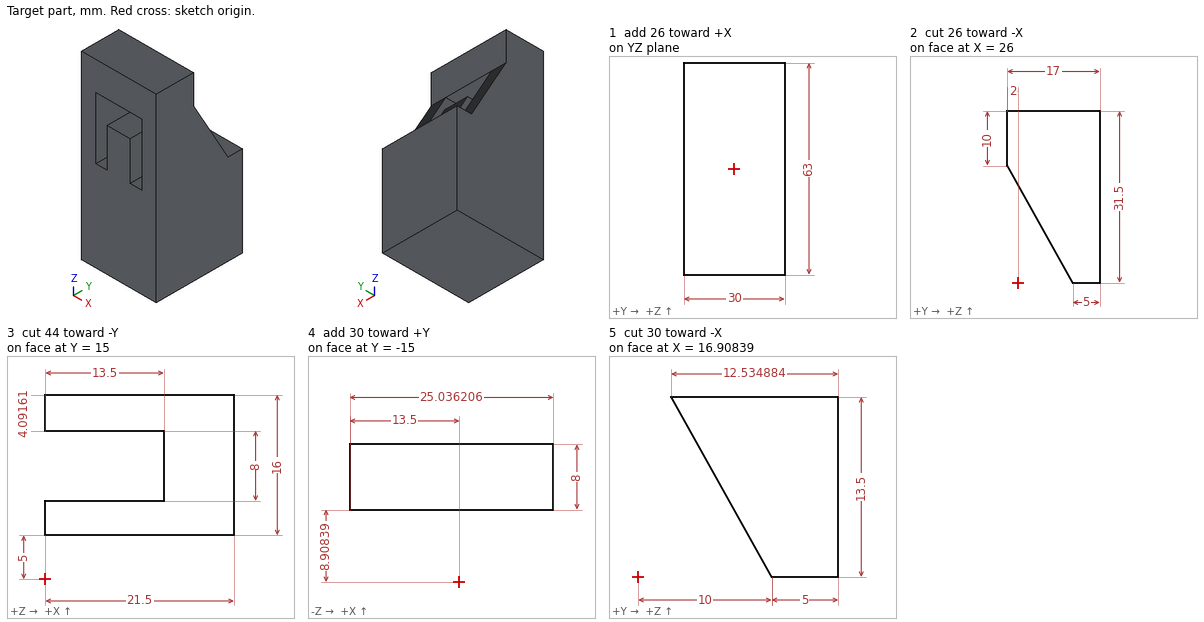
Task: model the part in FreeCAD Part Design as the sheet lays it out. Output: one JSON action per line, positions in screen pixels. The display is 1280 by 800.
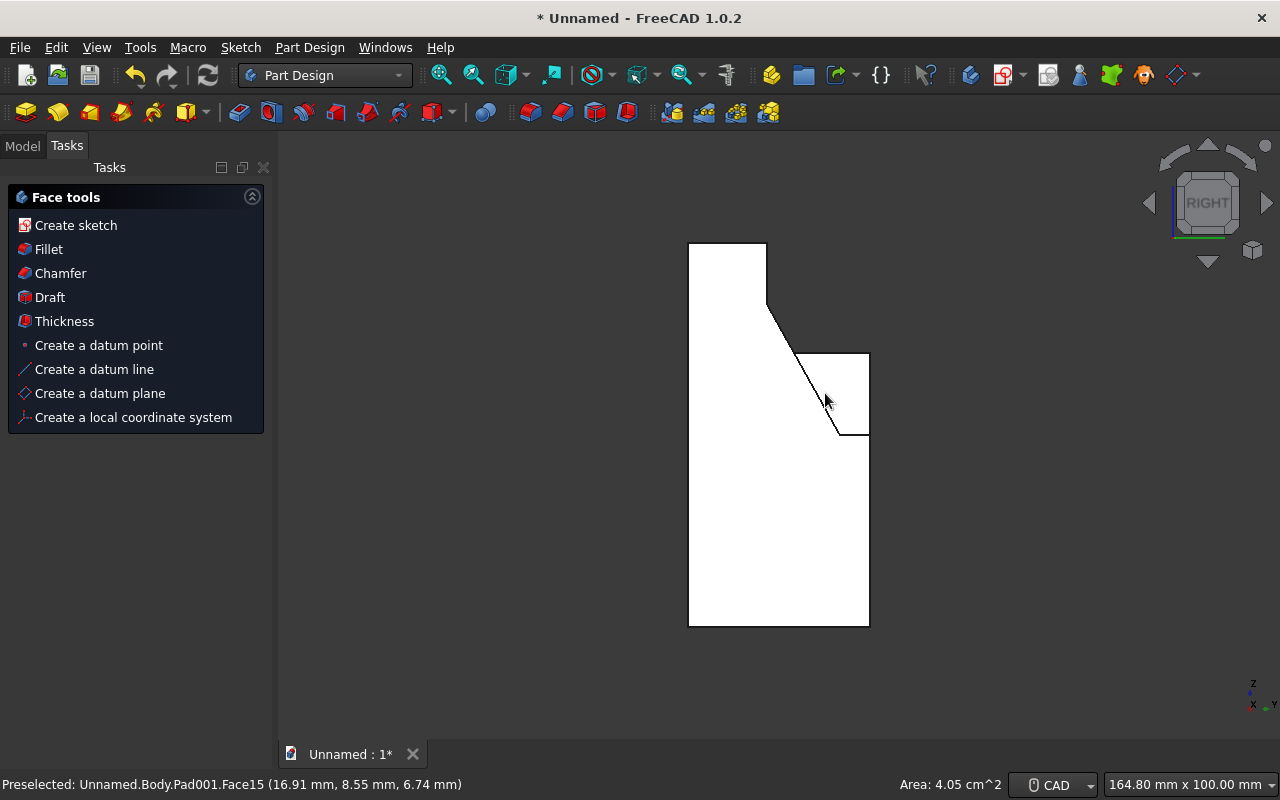
{"action": "left_click", "coordinate": [1004, 76]}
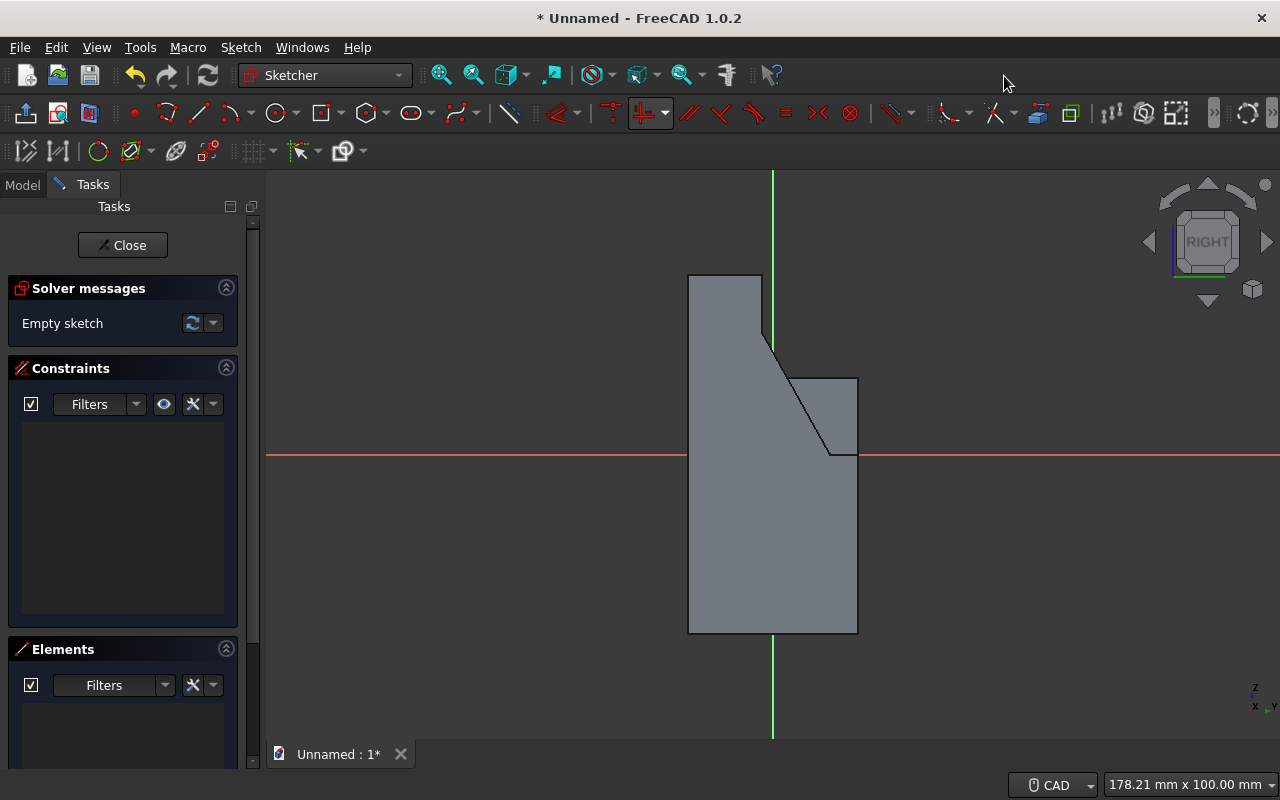
{"action": "scroll", "coordinate": [844, 406], "scroll_direction": "up", "scroll_amount": 8}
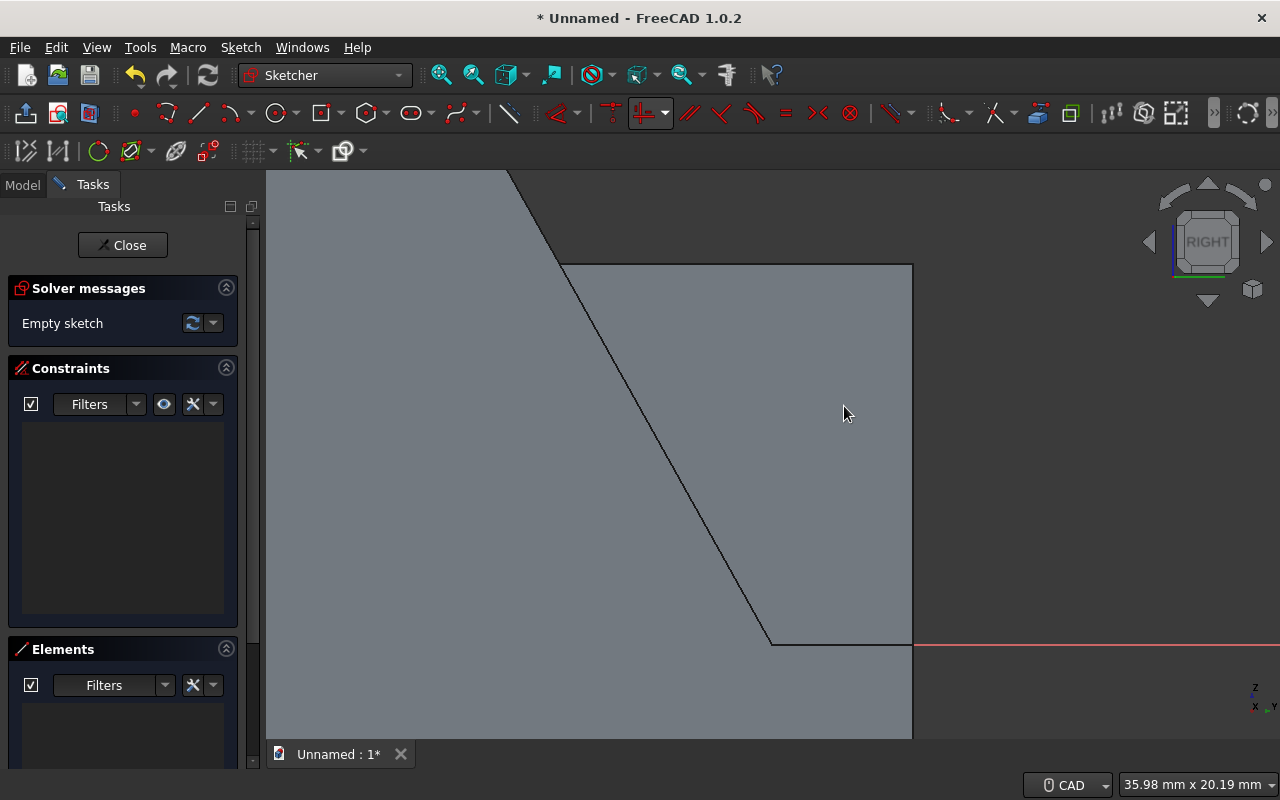
{"action": "left_click", "coordinate": [168, 114]}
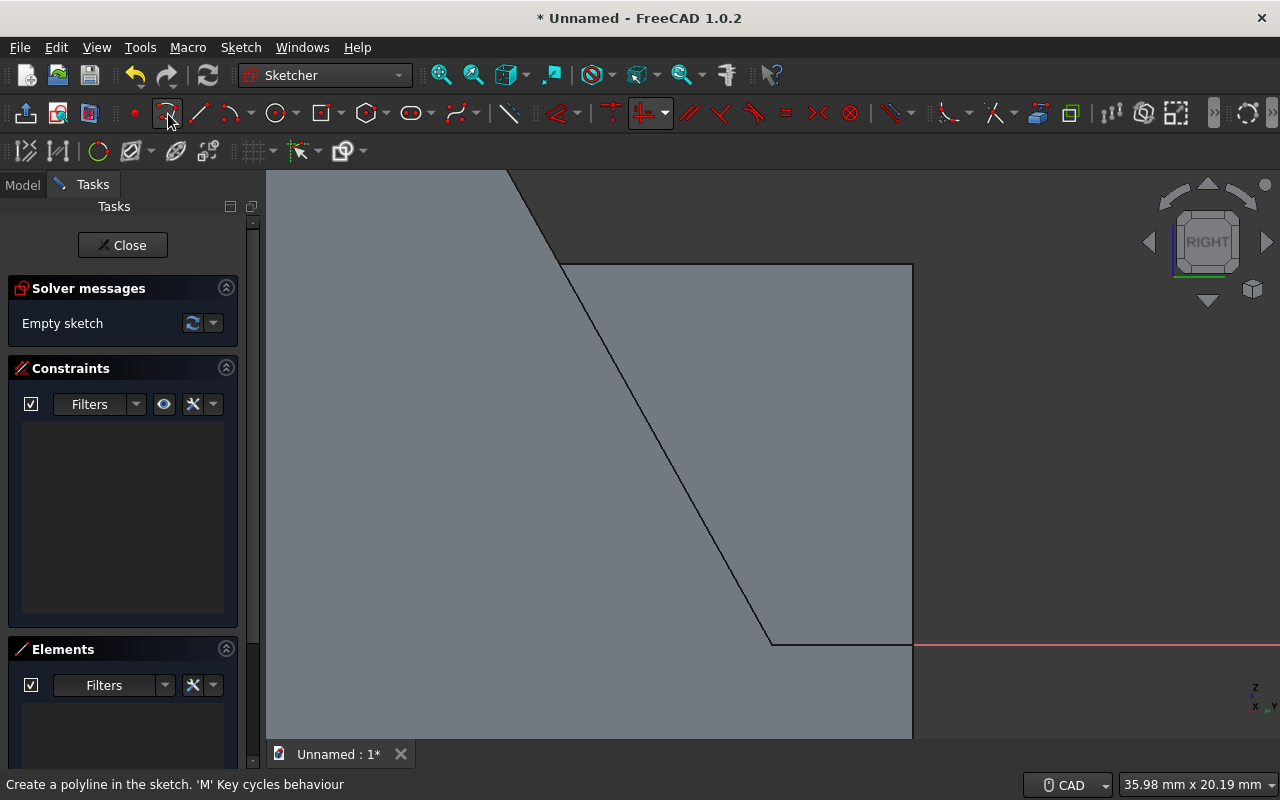
{"action": "left_click", "coordinate": [772, 645]}
{"action": "left_click", "coordinate": [913, 636]}
{"action": "left_click", "coordinate": [913, 264]}
{"action": "left_click", "coordinate": [560, 264]}
{"action": "left_click", "coordinate": [772, 645]}
{"action": "key", "text": "Escape"}
{"action": "key", "text": "Escape"}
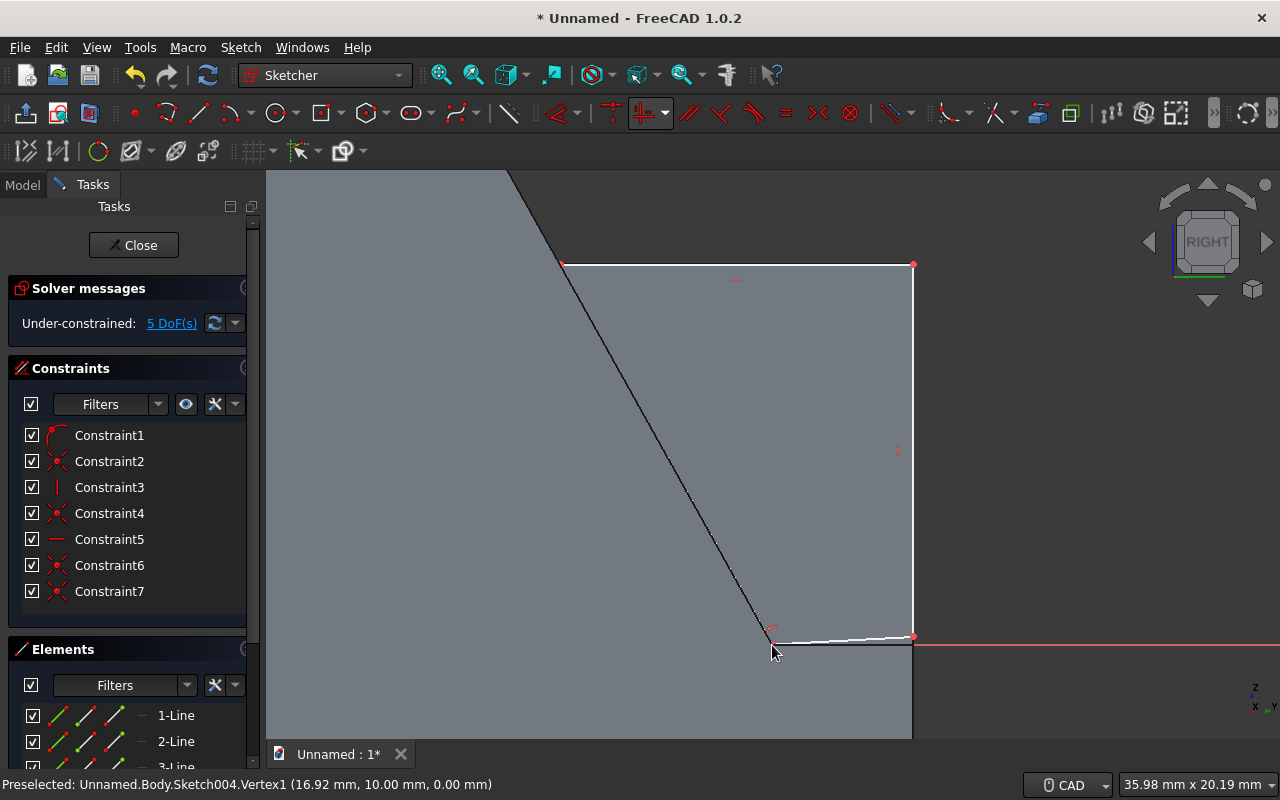
{"action": "left_click", "coordinate": [814, 642]}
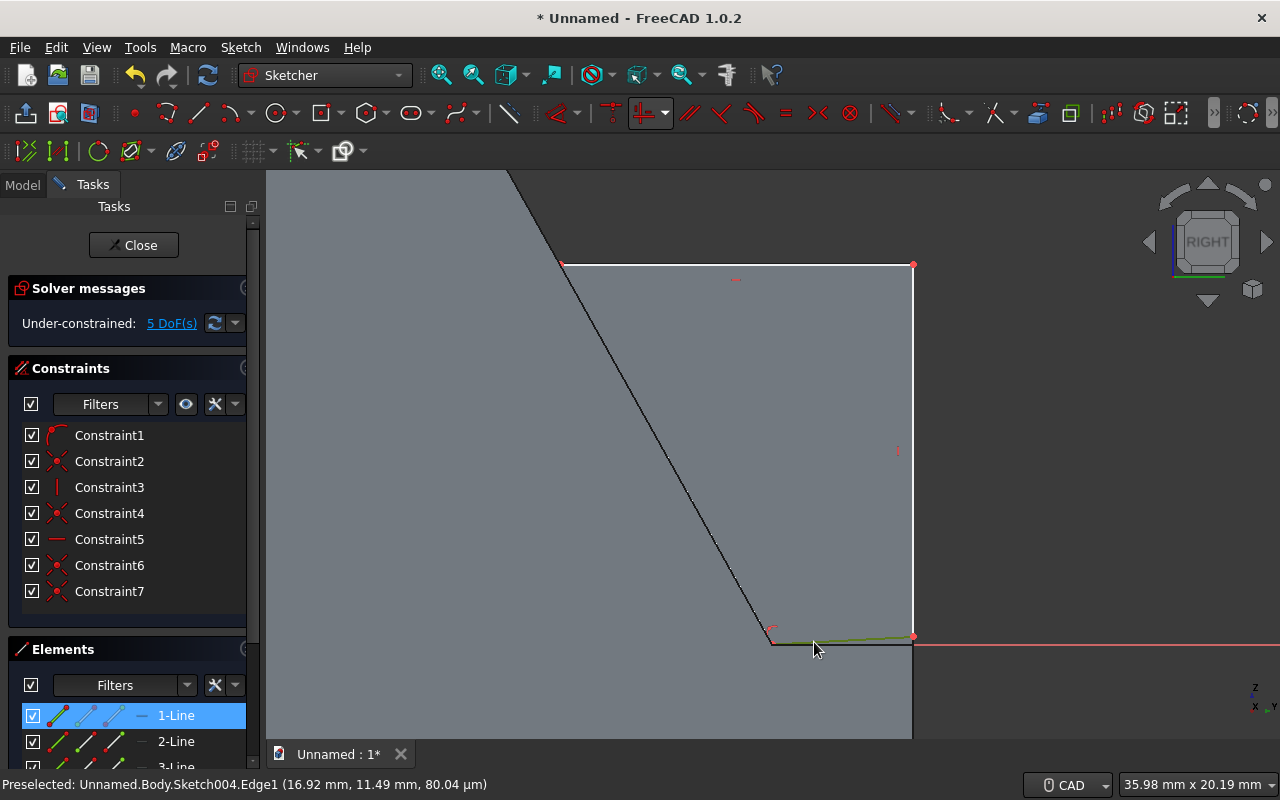
{"action": "left_click", "coordinate": [668, 114]}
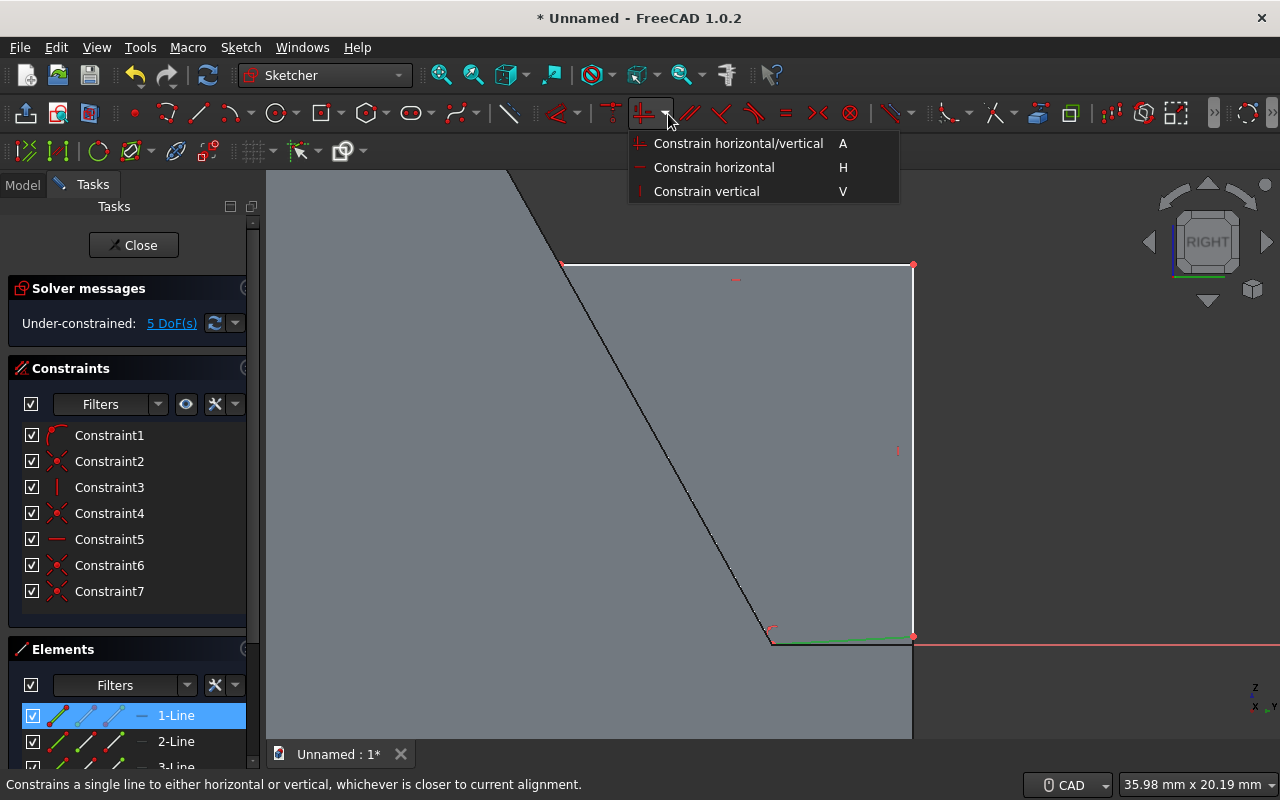
{"action": "left_click", "coordinate": [764, 167]}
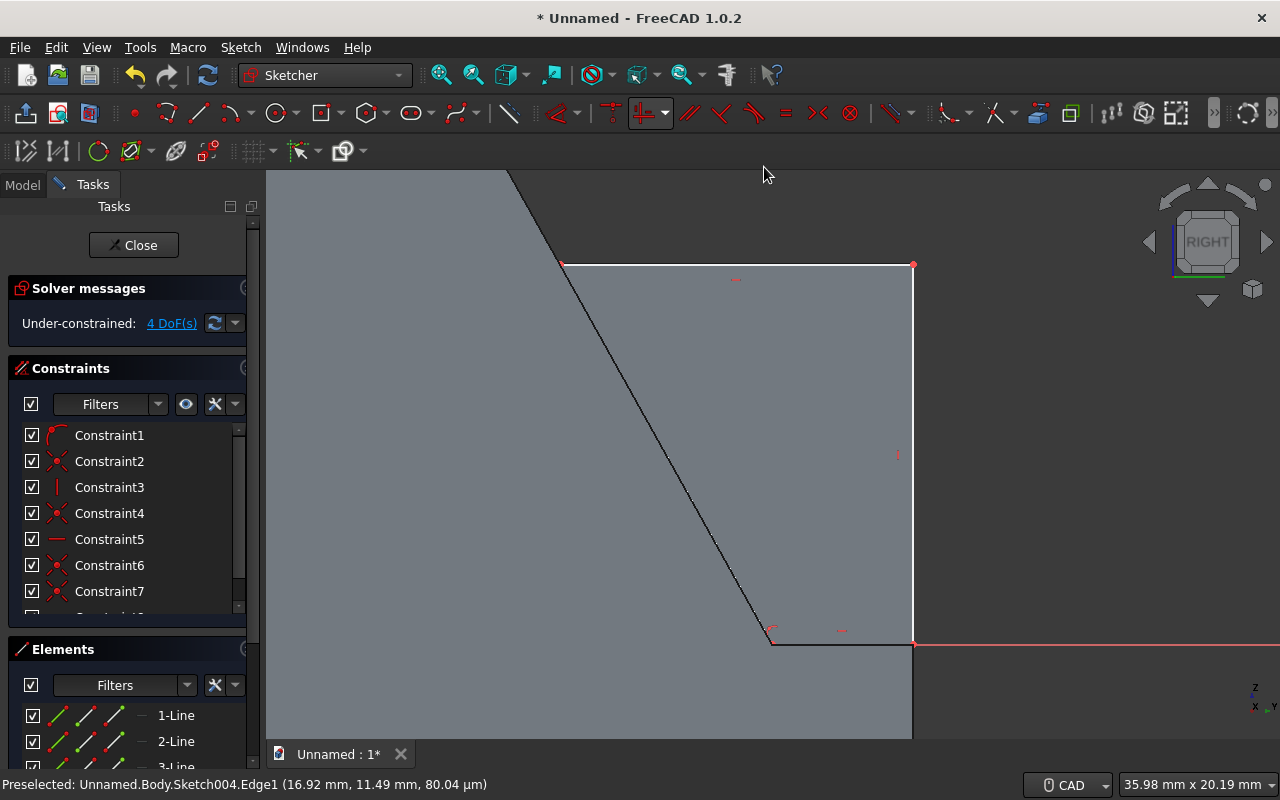
{"action": "left_click", "coordinate": [556, 114]}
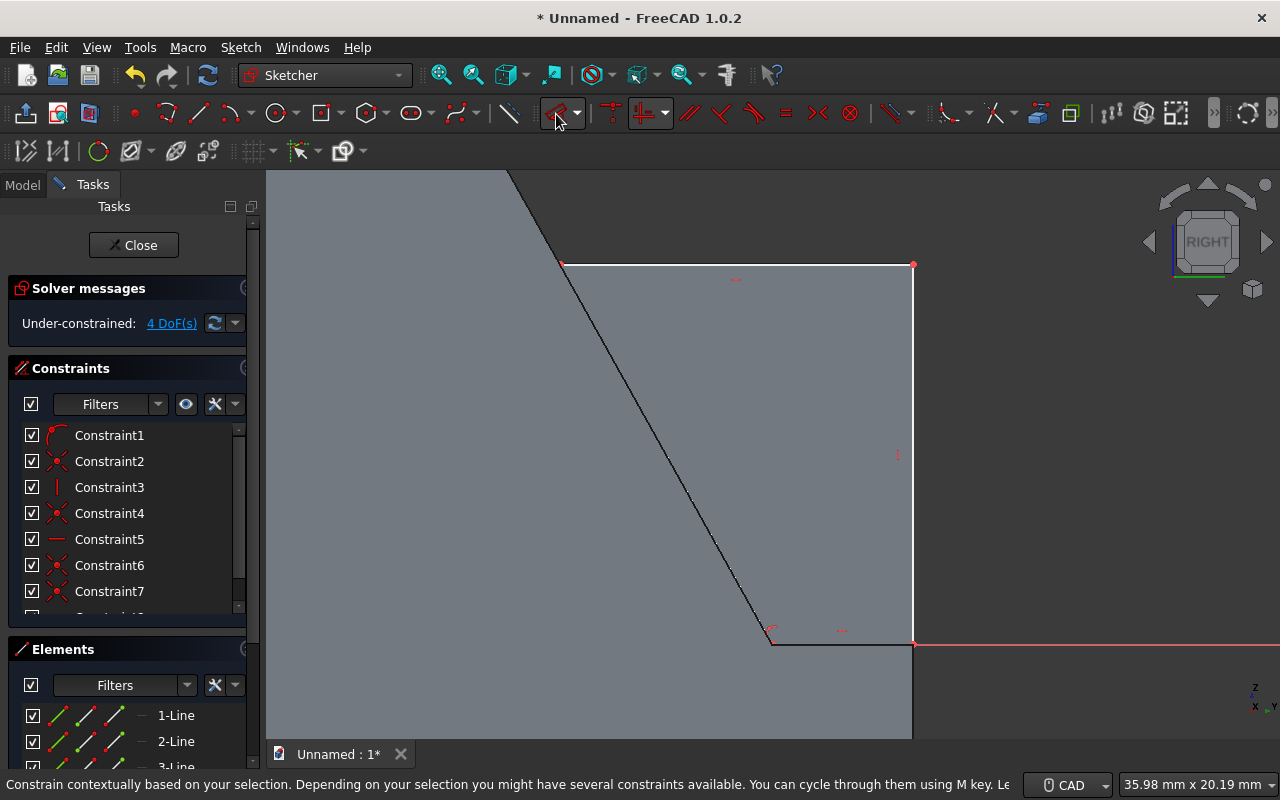
{"action": "left_click", "coordinate": [814, 645]}
{"action": "left_click", "coordinate": [843, 679]}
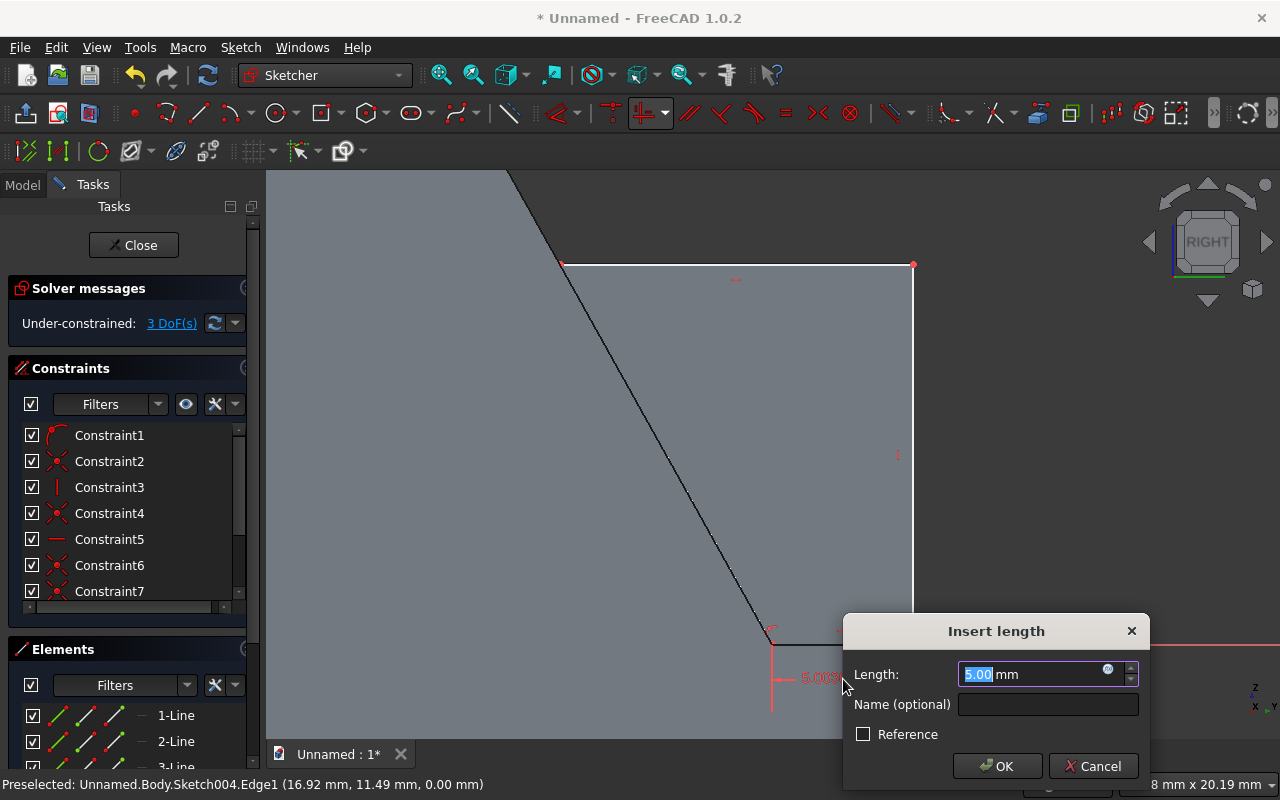
{"action": "type", "text": "5"}
{"action": "key", "text": "Return"}